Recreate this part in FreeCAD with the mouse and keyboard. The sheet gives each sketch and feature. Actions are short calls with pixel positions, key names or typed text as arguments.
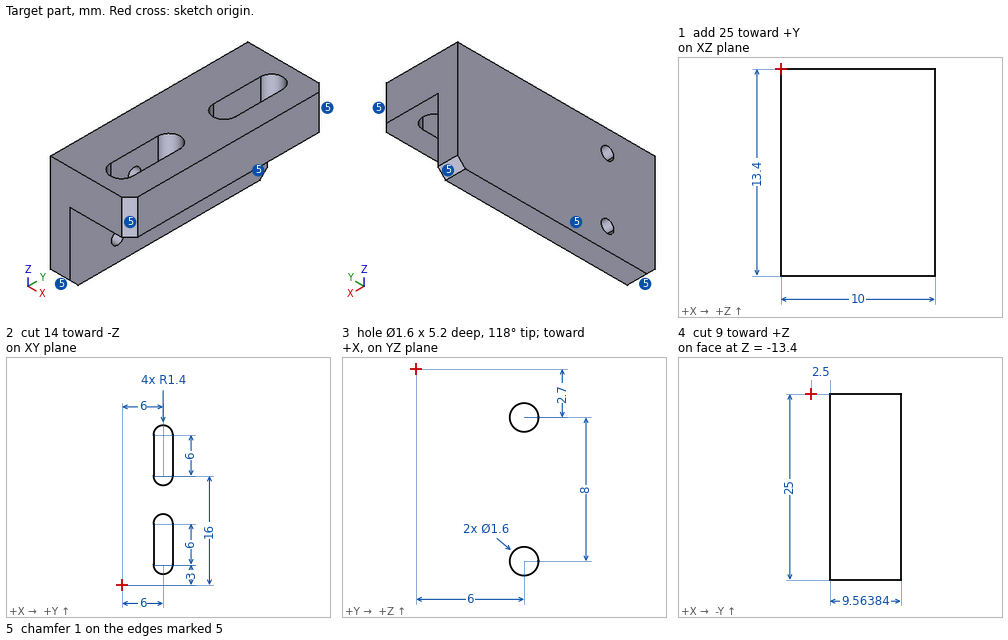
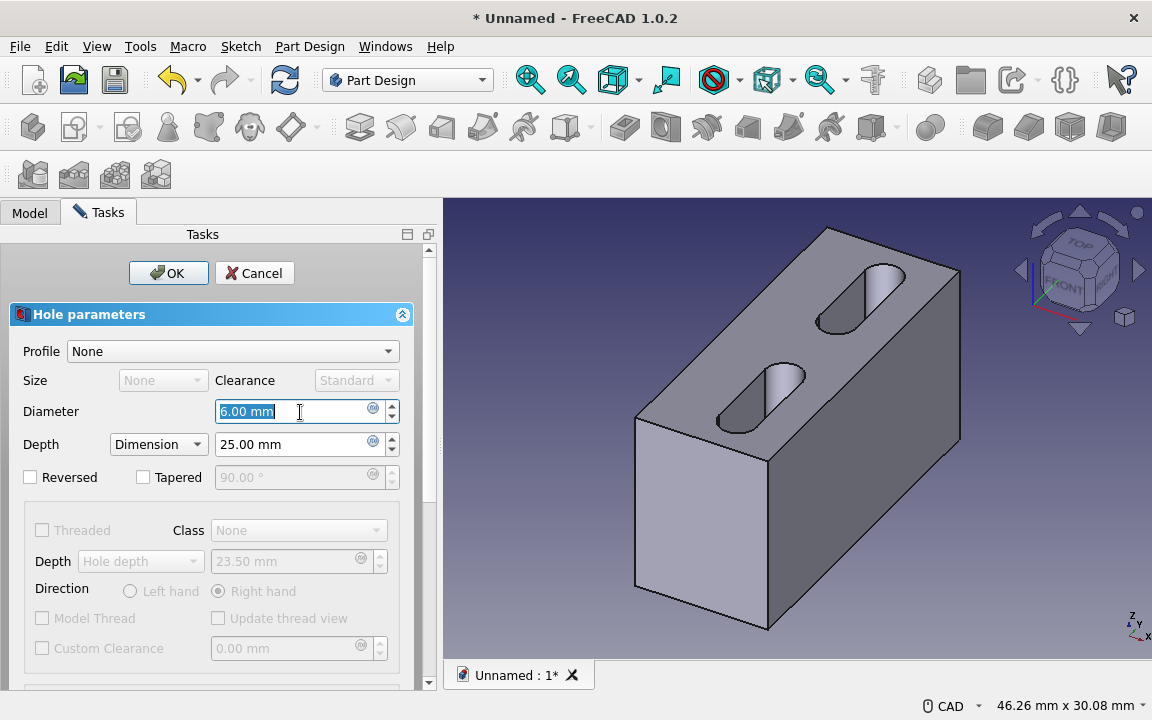
text(1.6)
key(Tab)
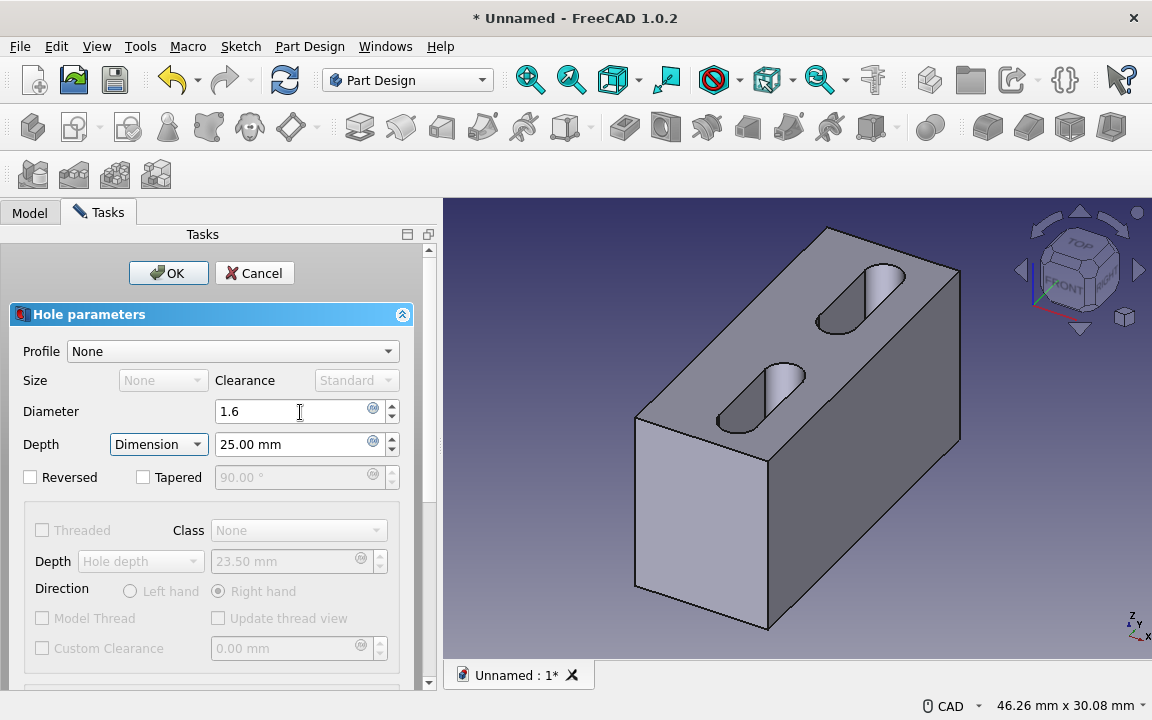
triple_click(300, 444)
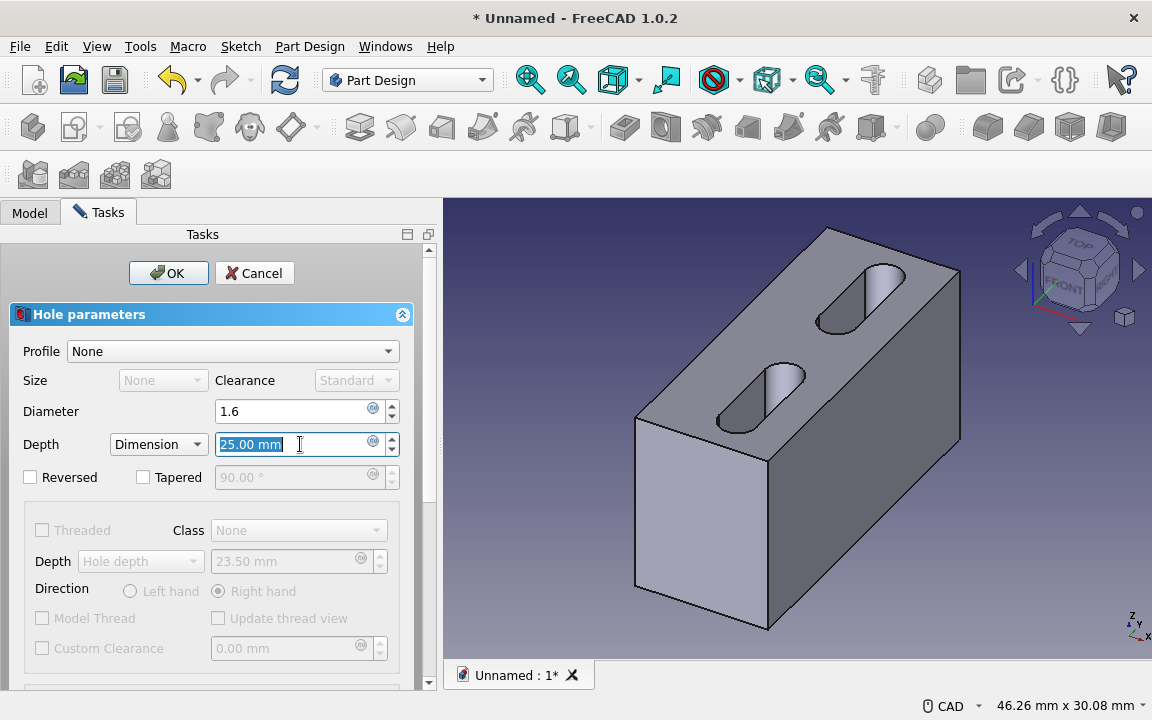
text(5.2)
key(Tab)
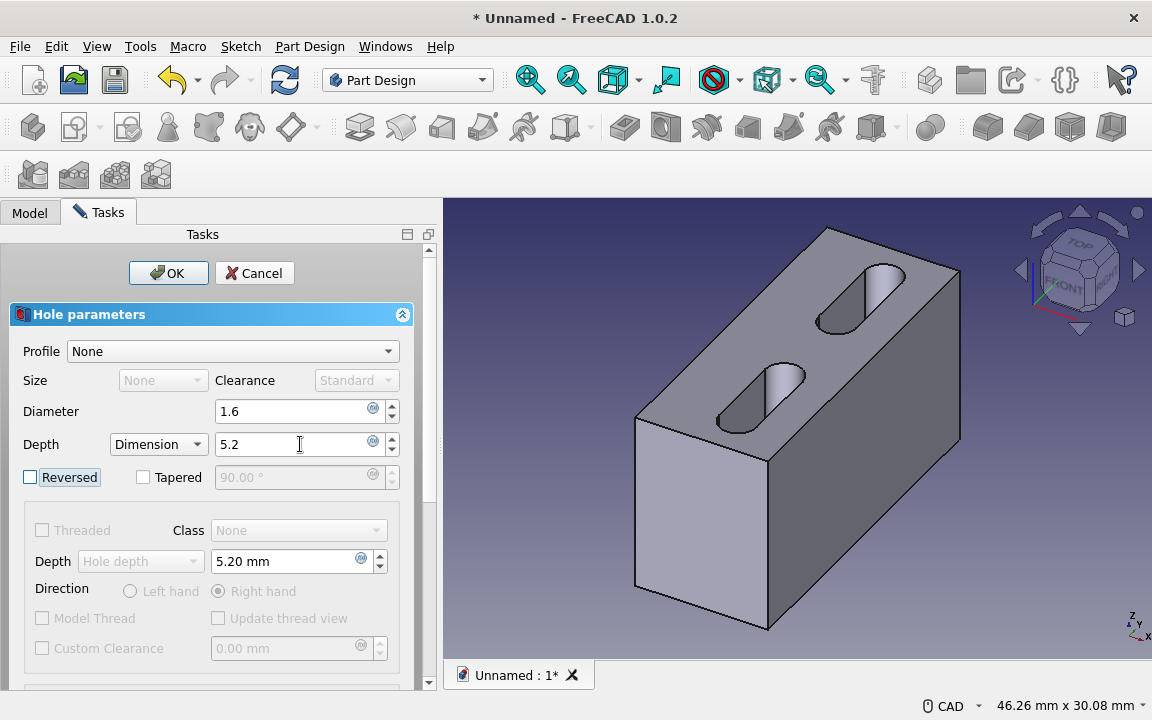
click(31, 477)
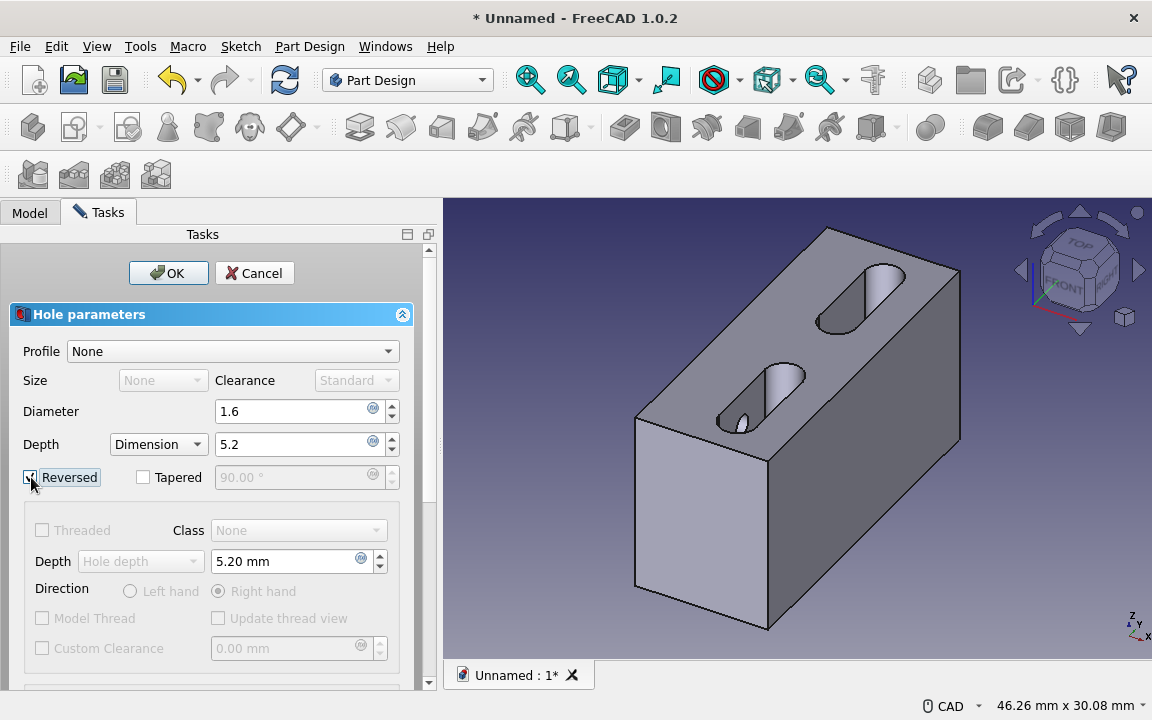
click(169, 273)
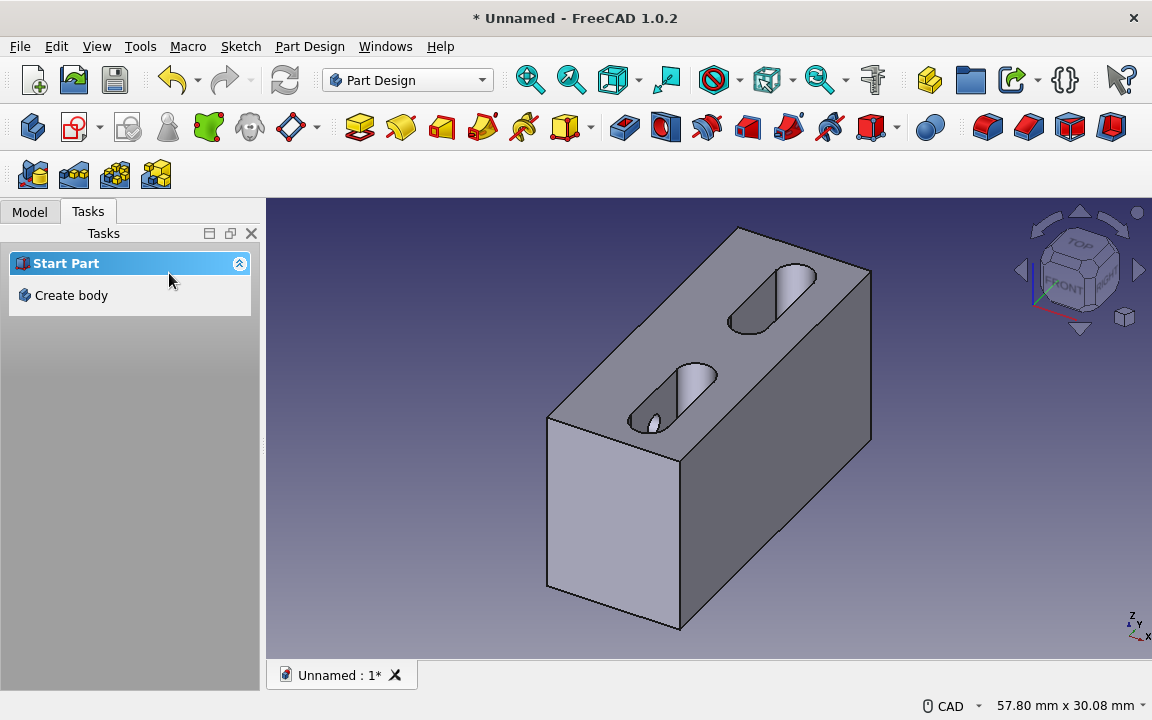
key(5)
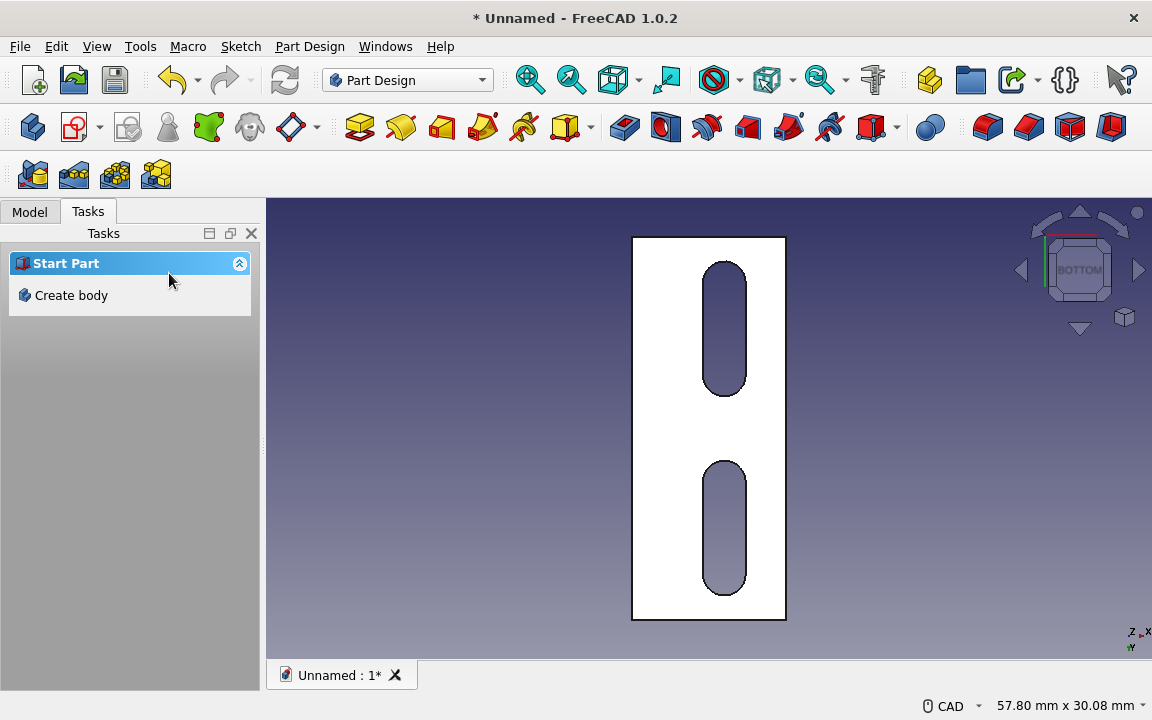
click(687, 427)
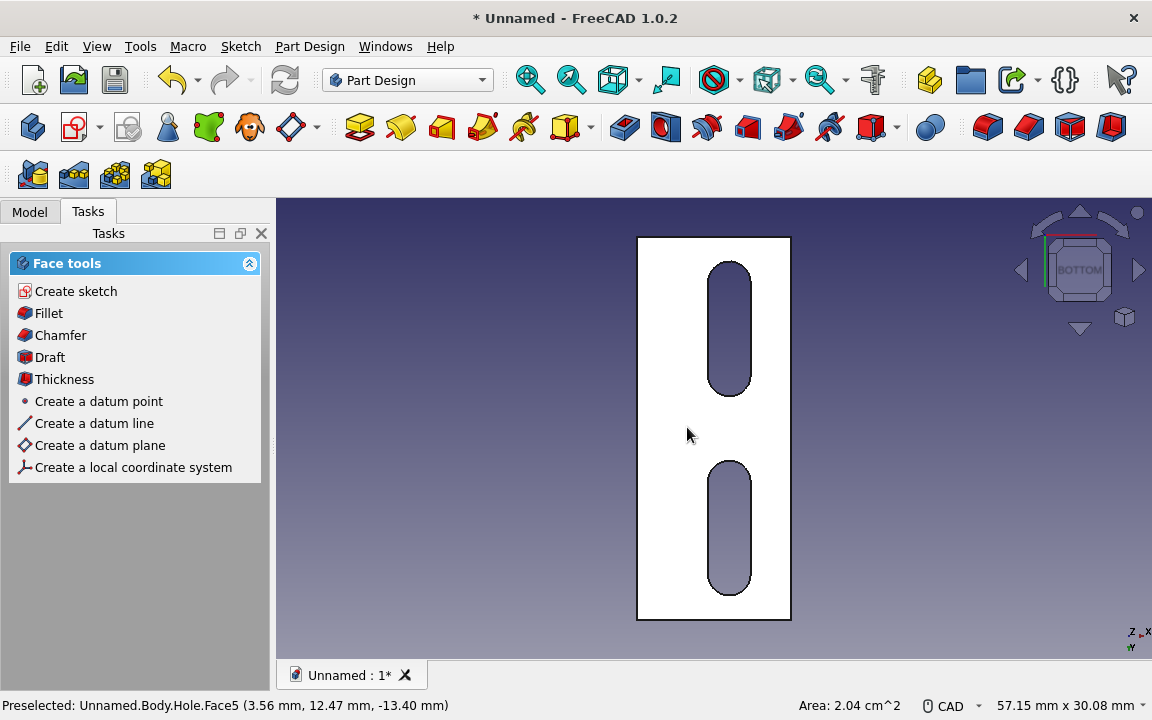
click(74, 128)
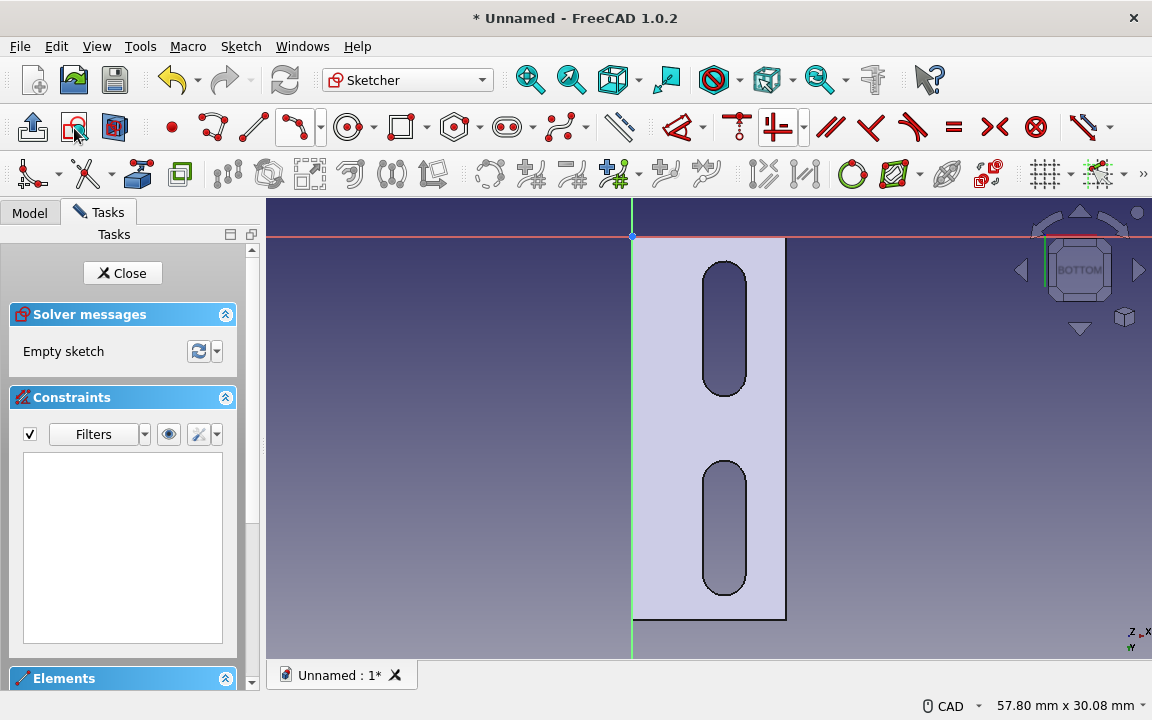
scroll(294, 429, down, 1)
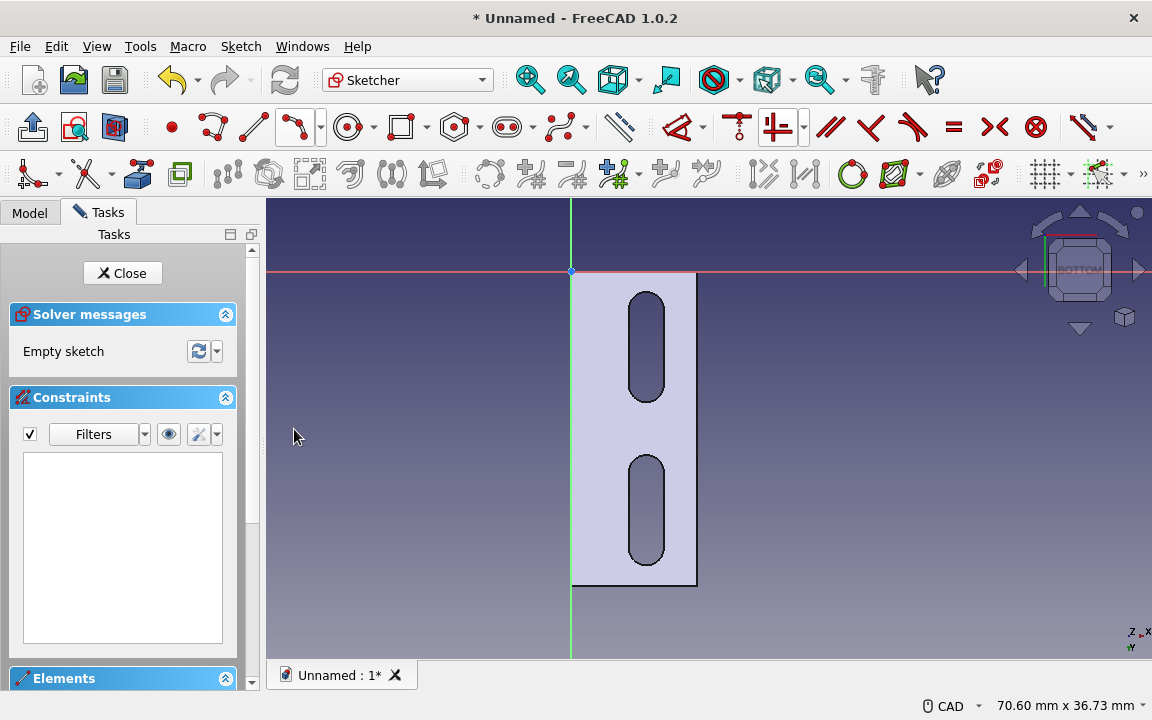
key(g)
key(r)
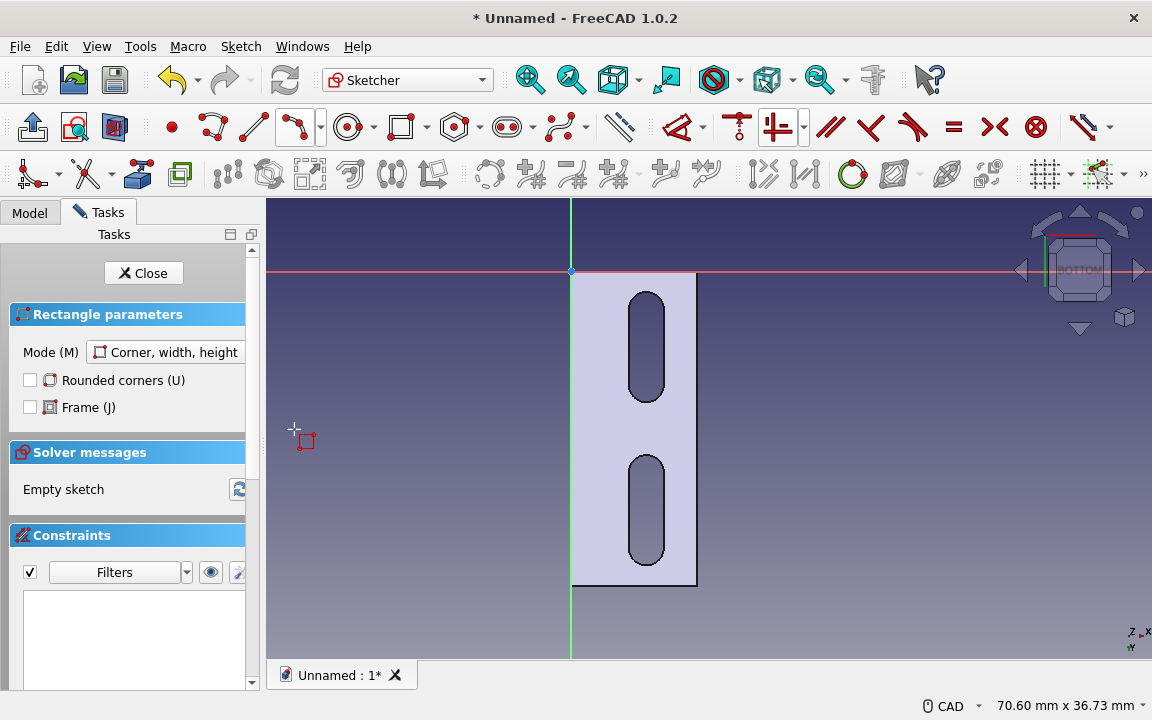
click(602, 272)
click(722, 586)
key(Escape)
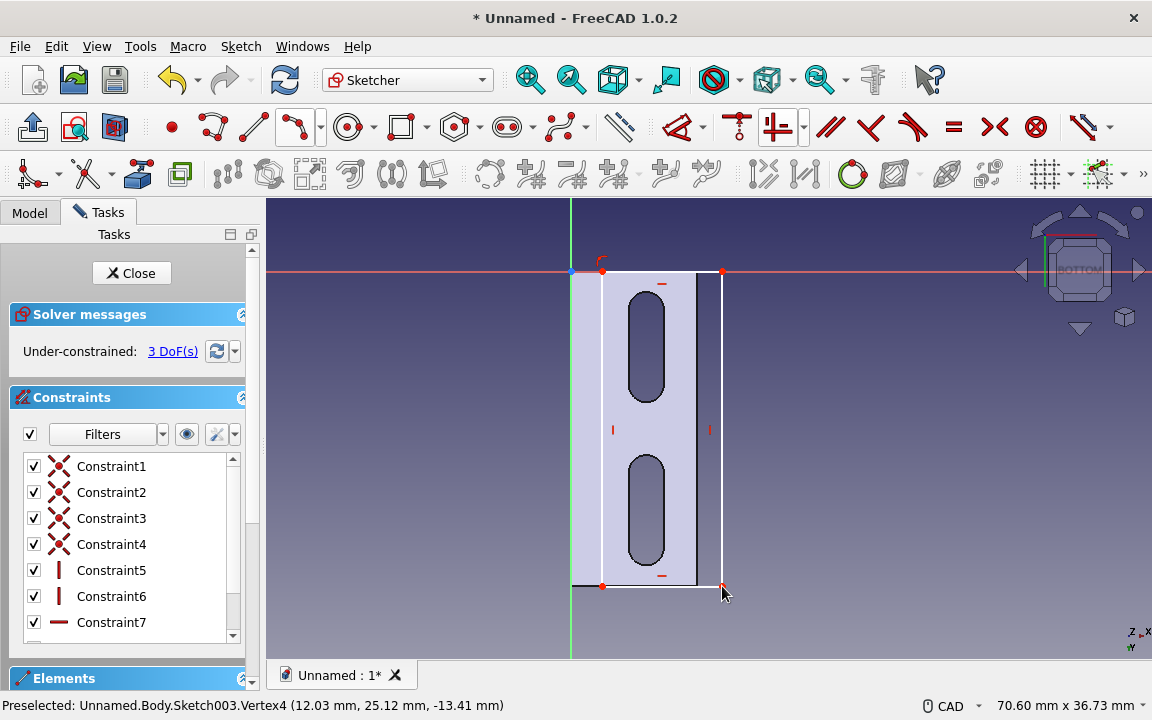
key(d)